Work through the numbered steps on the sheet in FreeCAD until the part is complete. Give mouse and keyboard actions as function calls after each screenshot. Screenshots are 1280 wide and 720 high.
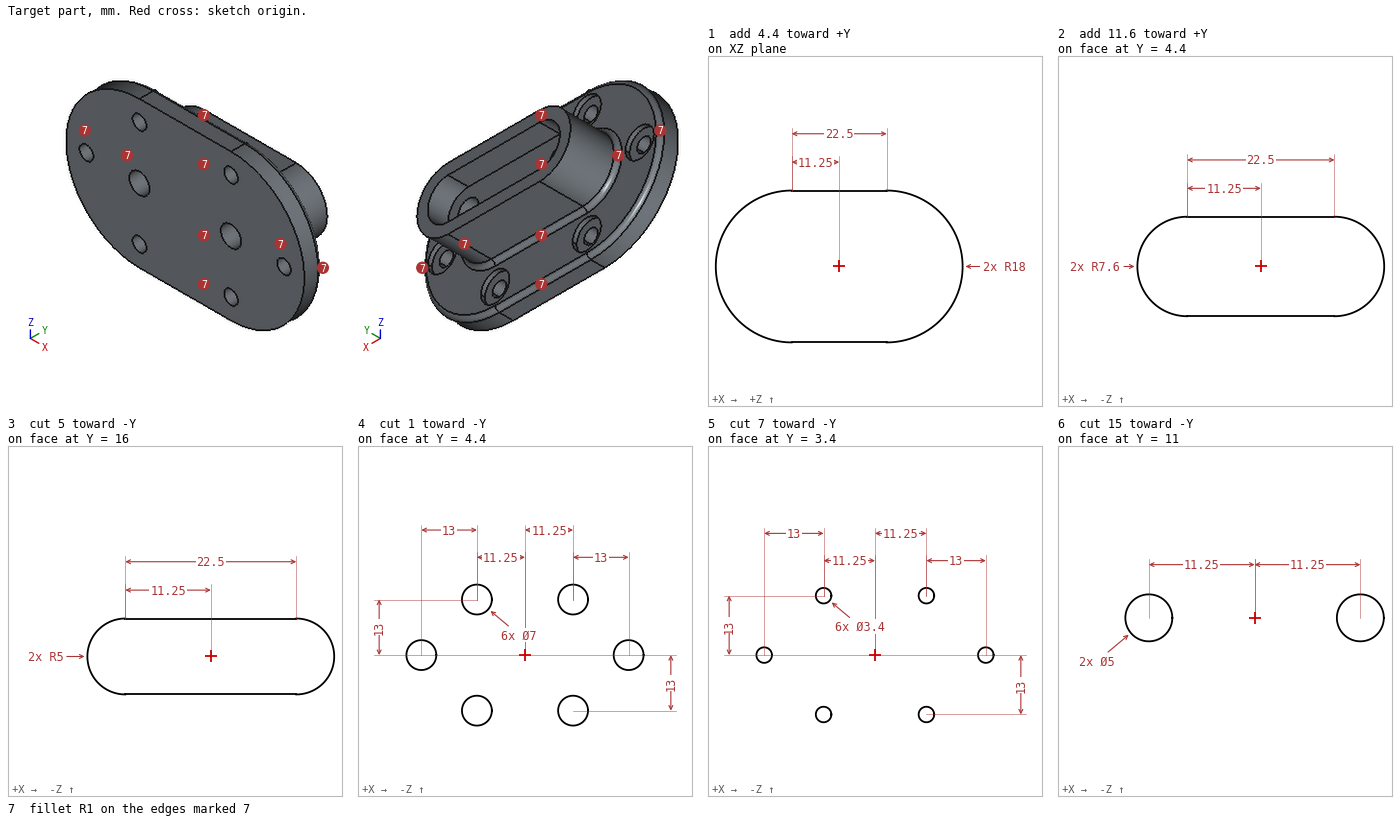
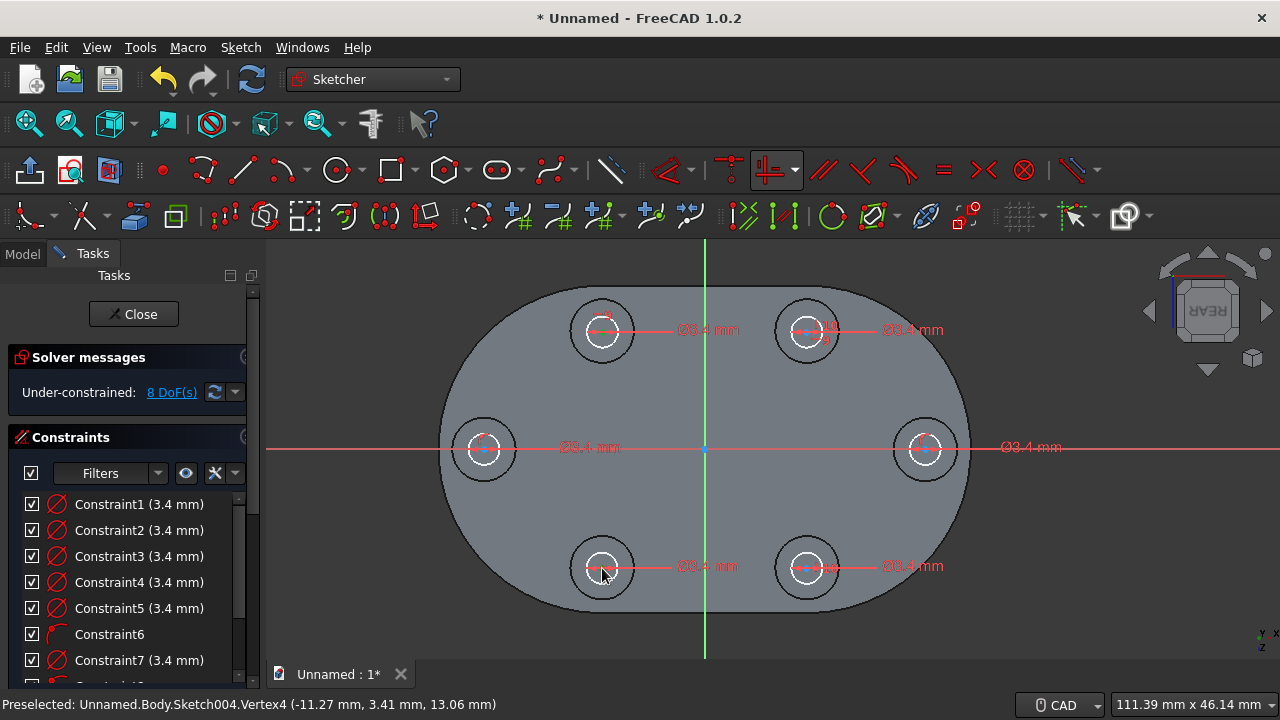
key(v)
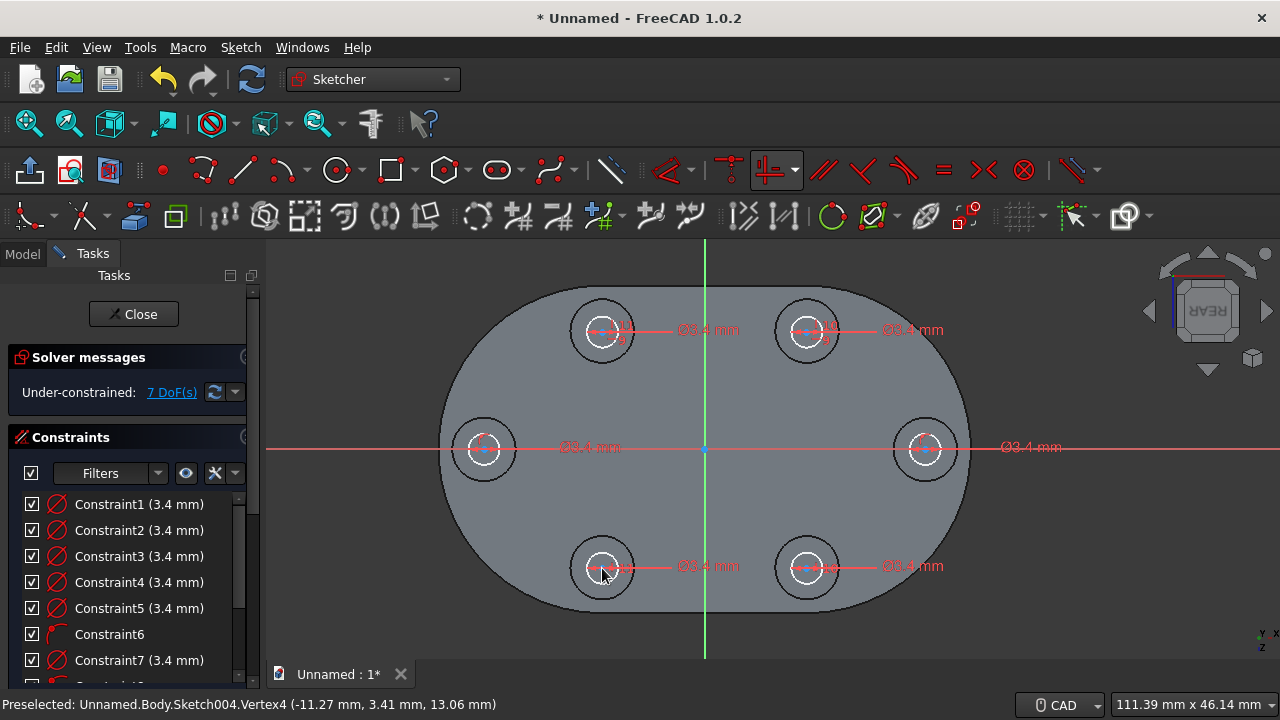
click(807, 568)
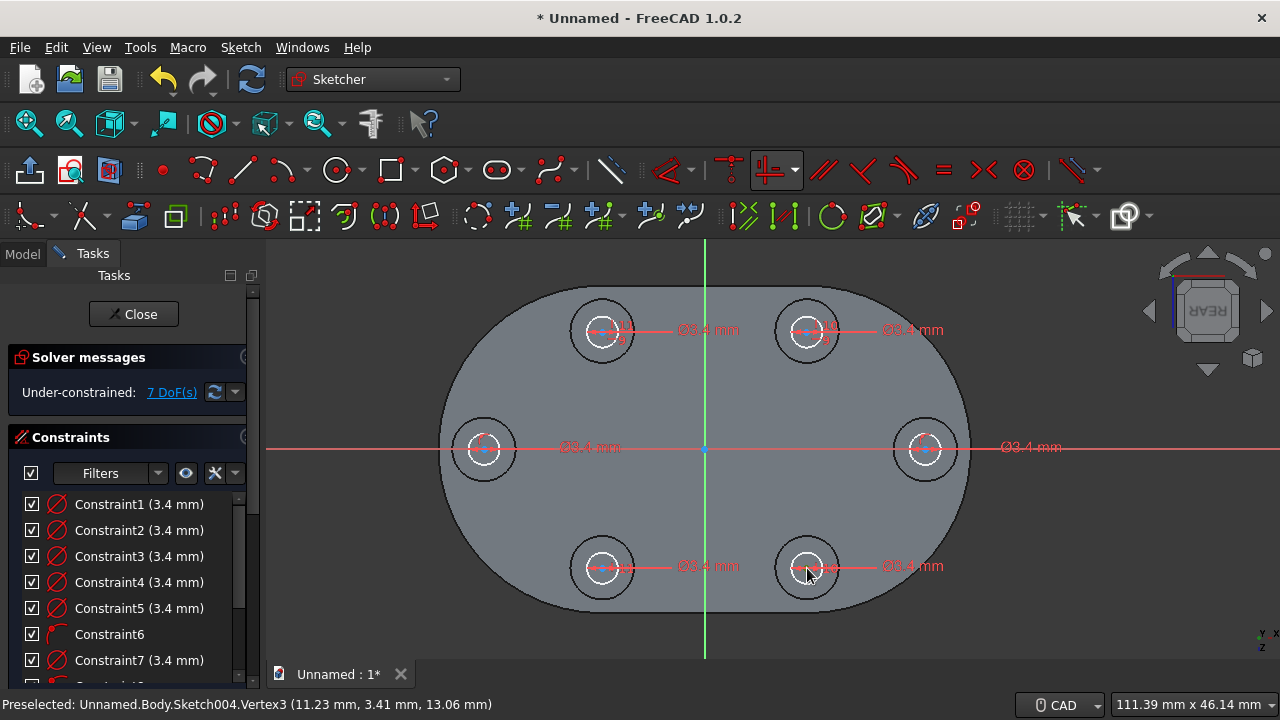
click(602, 568)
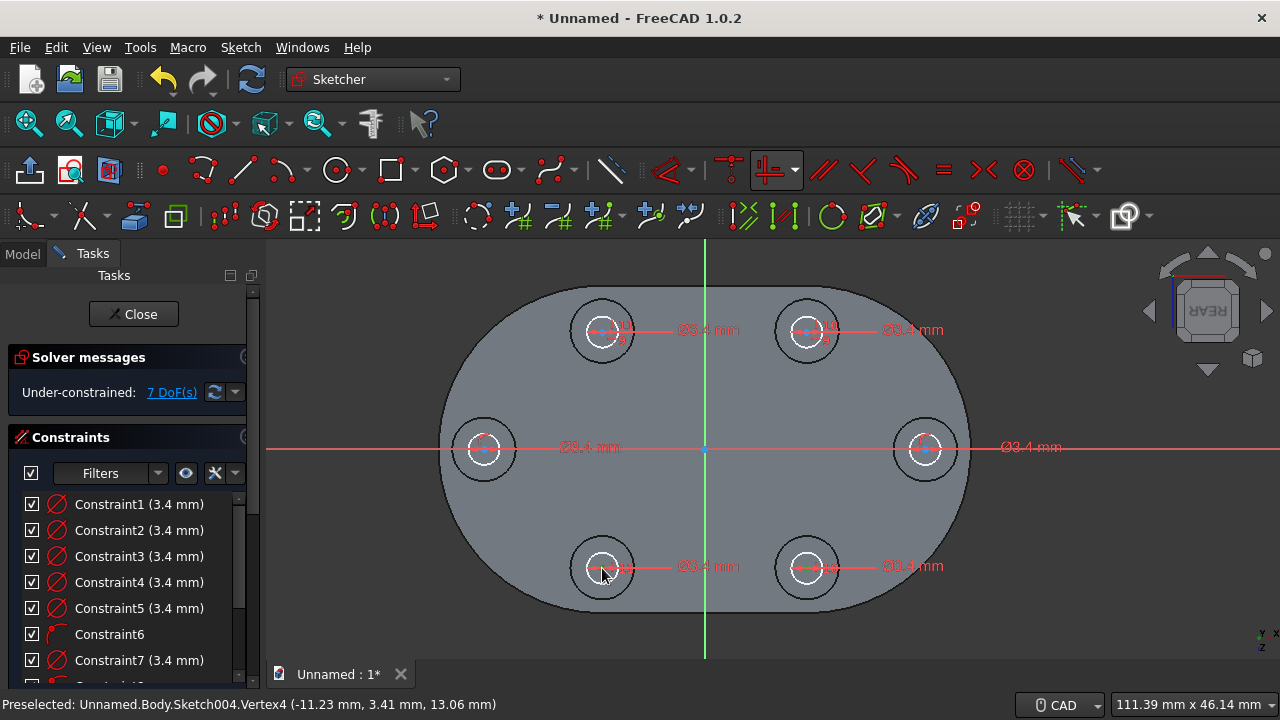
click(798, 170)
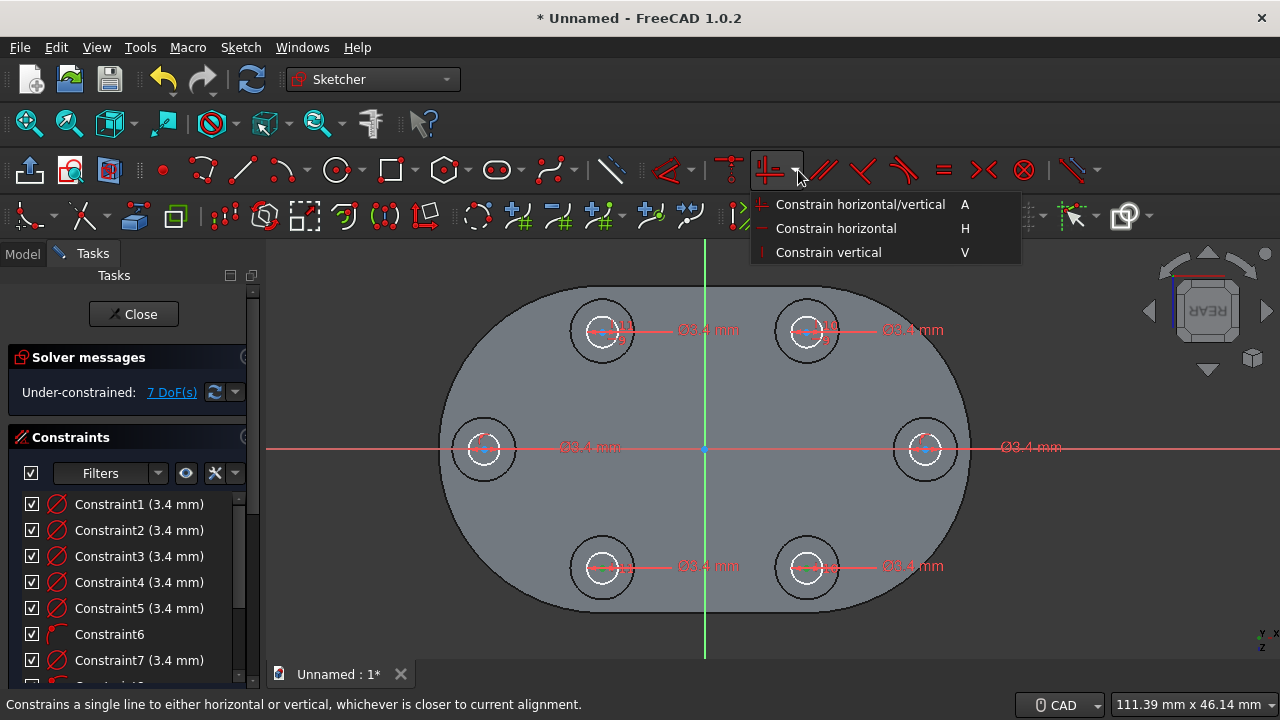
click(886, 228)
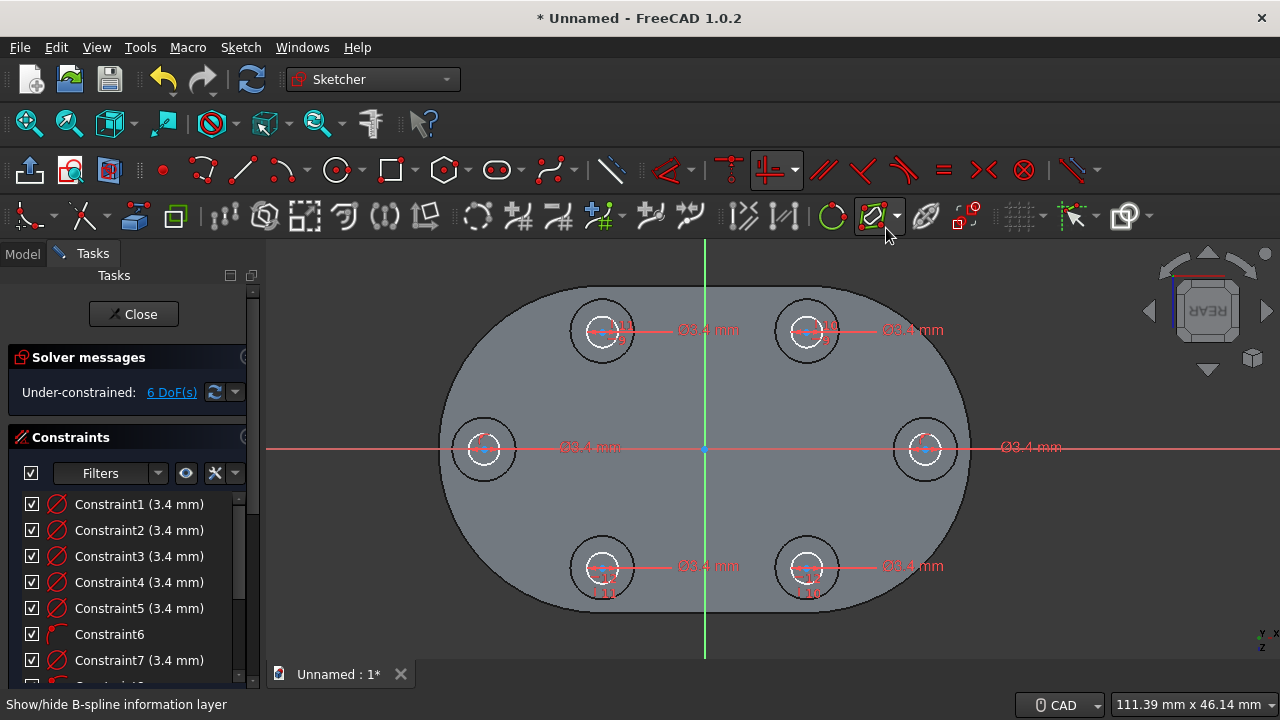
click(666, 170)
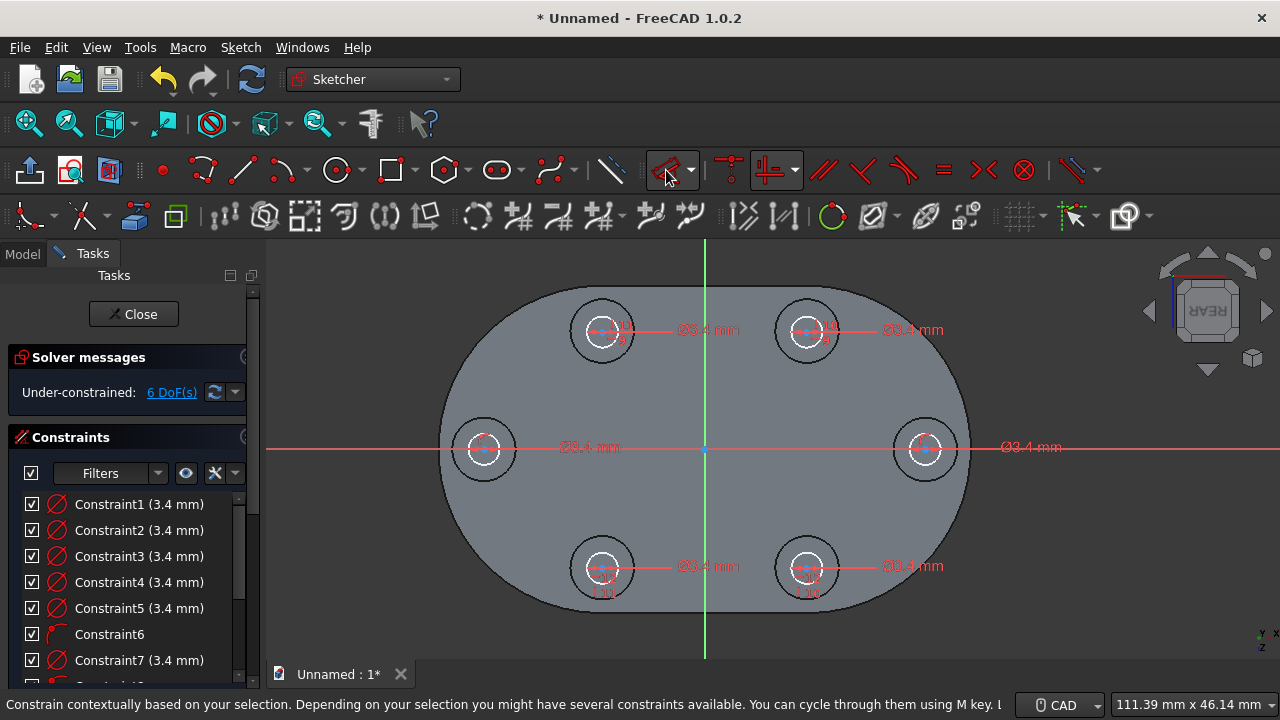
click(602, 332)
click(568, 391)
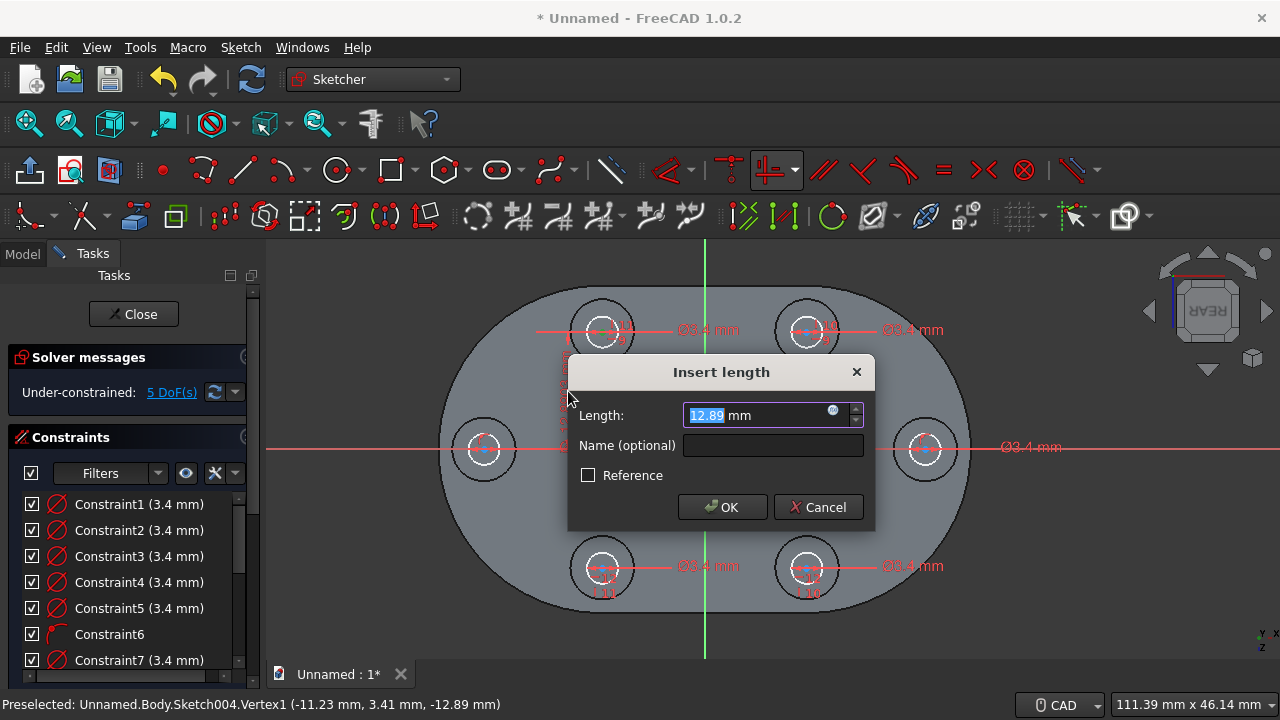
text(13)
key(Return)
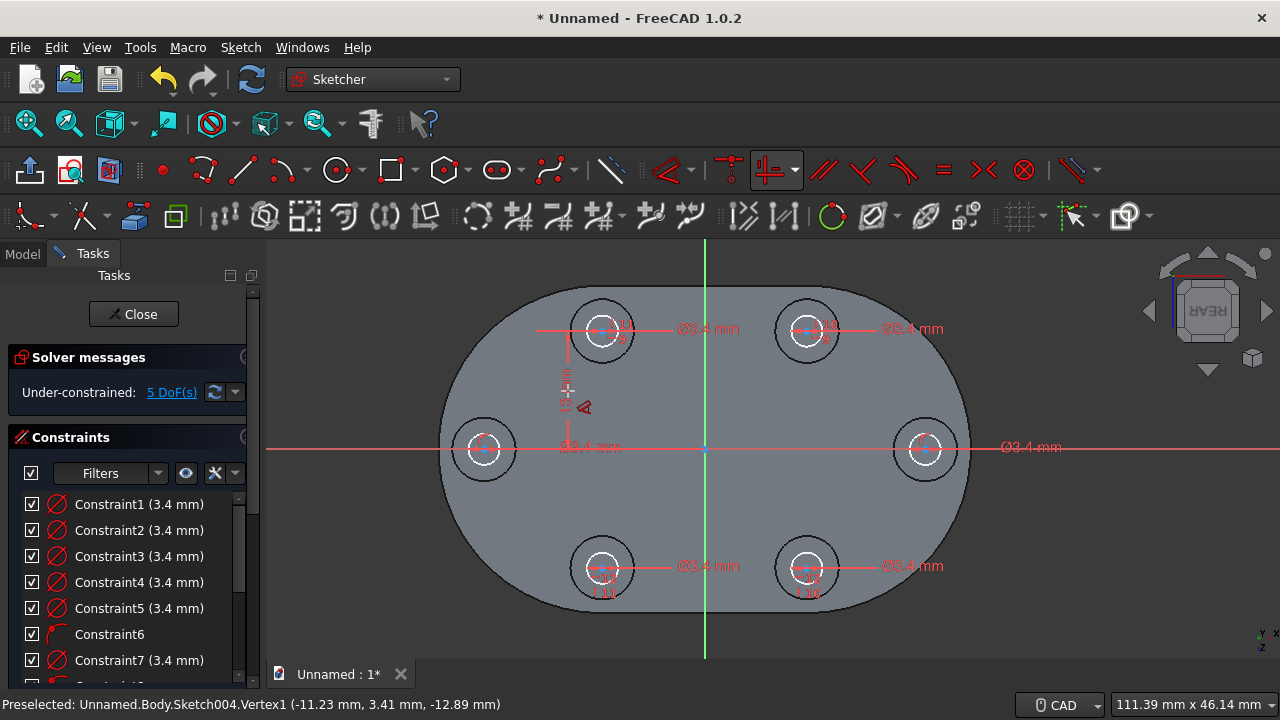
click(807, 568)
click(841, 509)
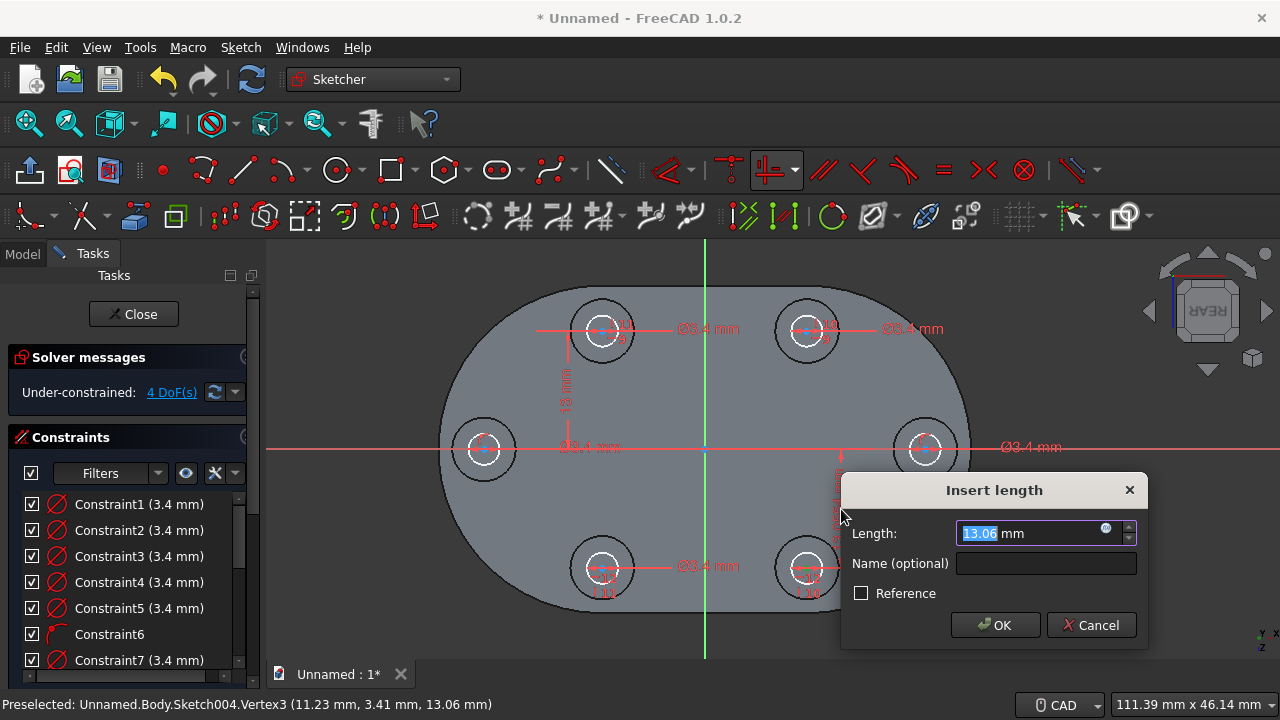
text(13)
key(Return)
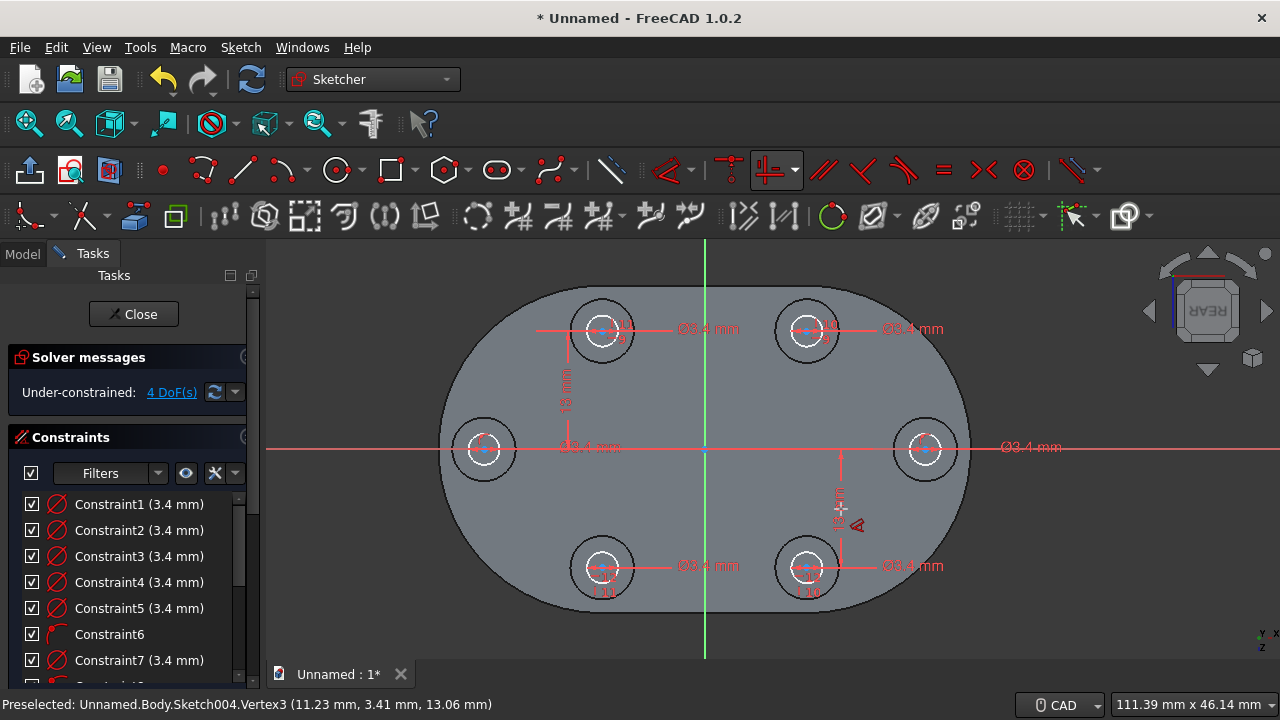
click(602, 331)